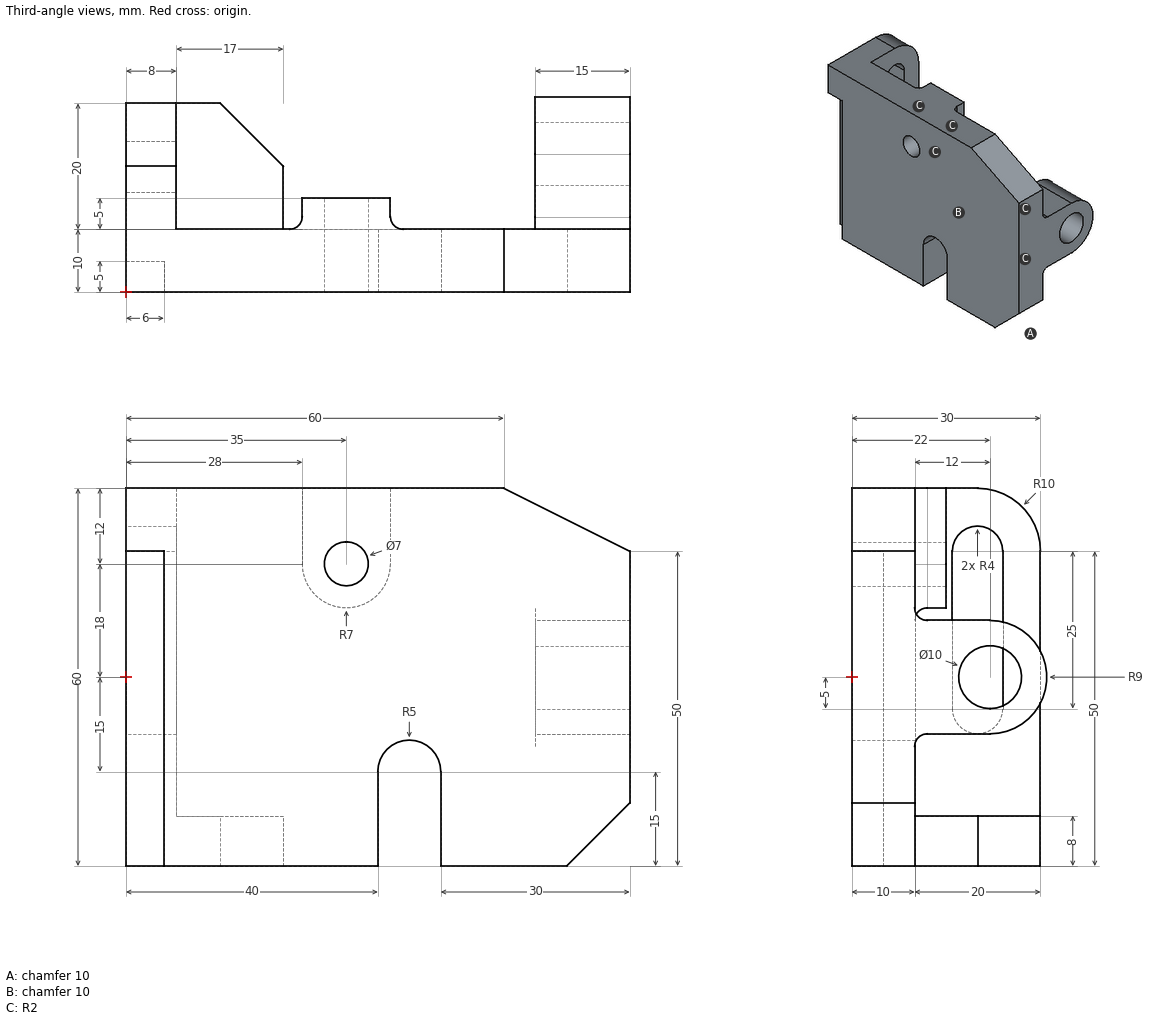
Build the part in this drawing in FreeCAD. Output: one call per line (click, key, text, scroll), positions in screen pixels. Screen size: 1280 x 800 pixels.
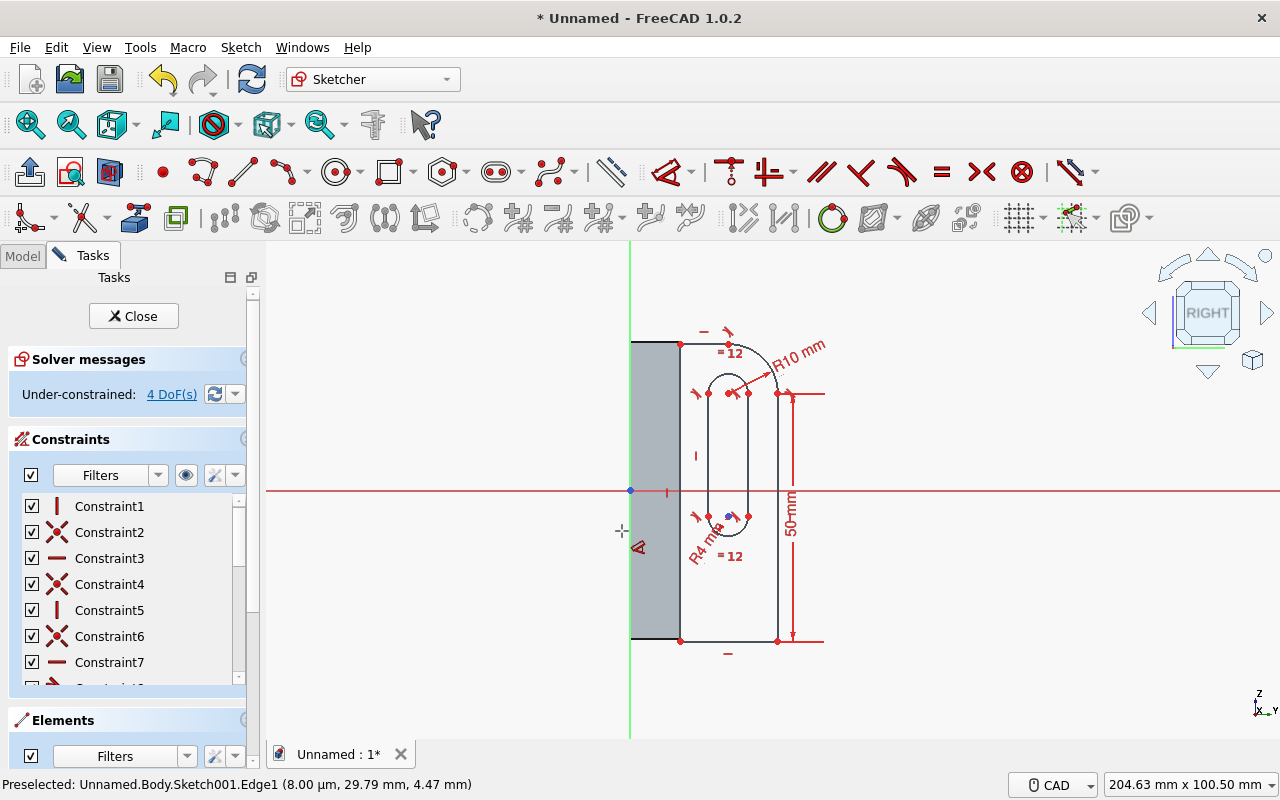
click(749, 642)
click(729, 676)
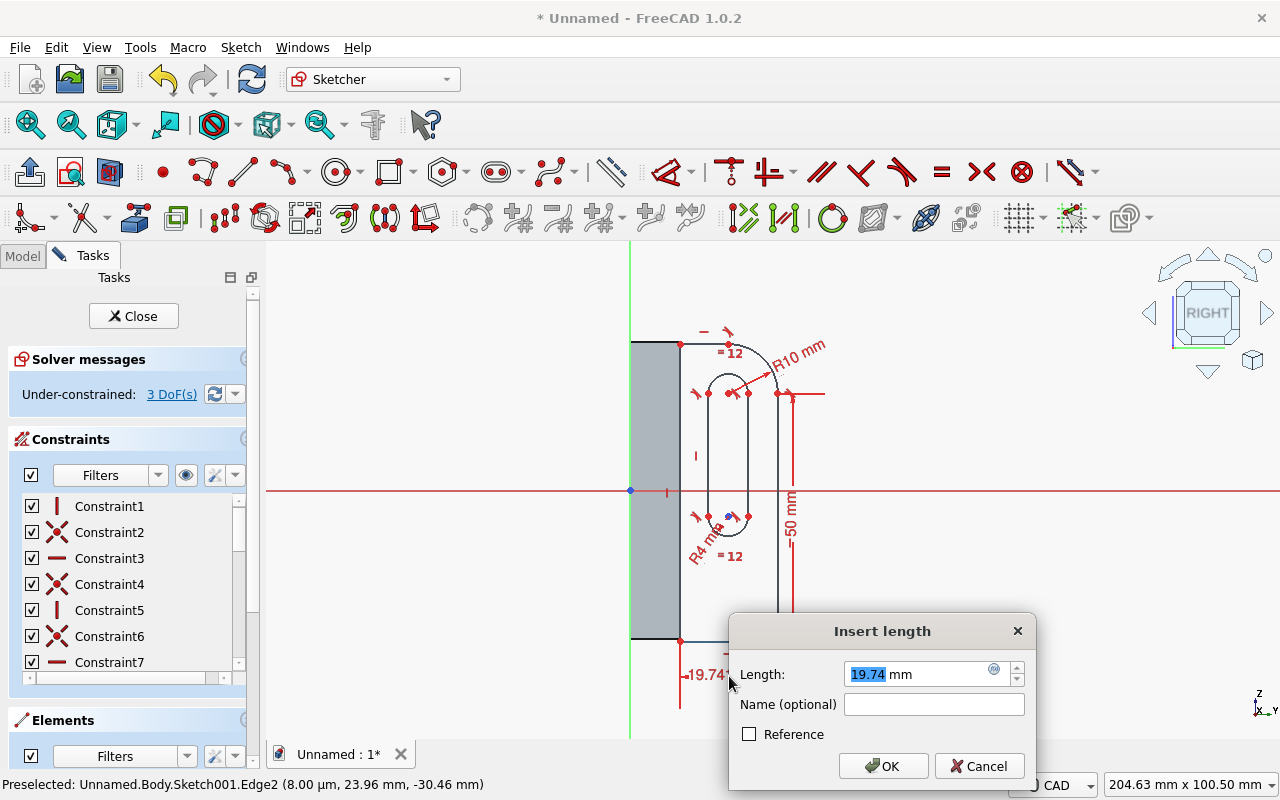
text(20)
key(Return)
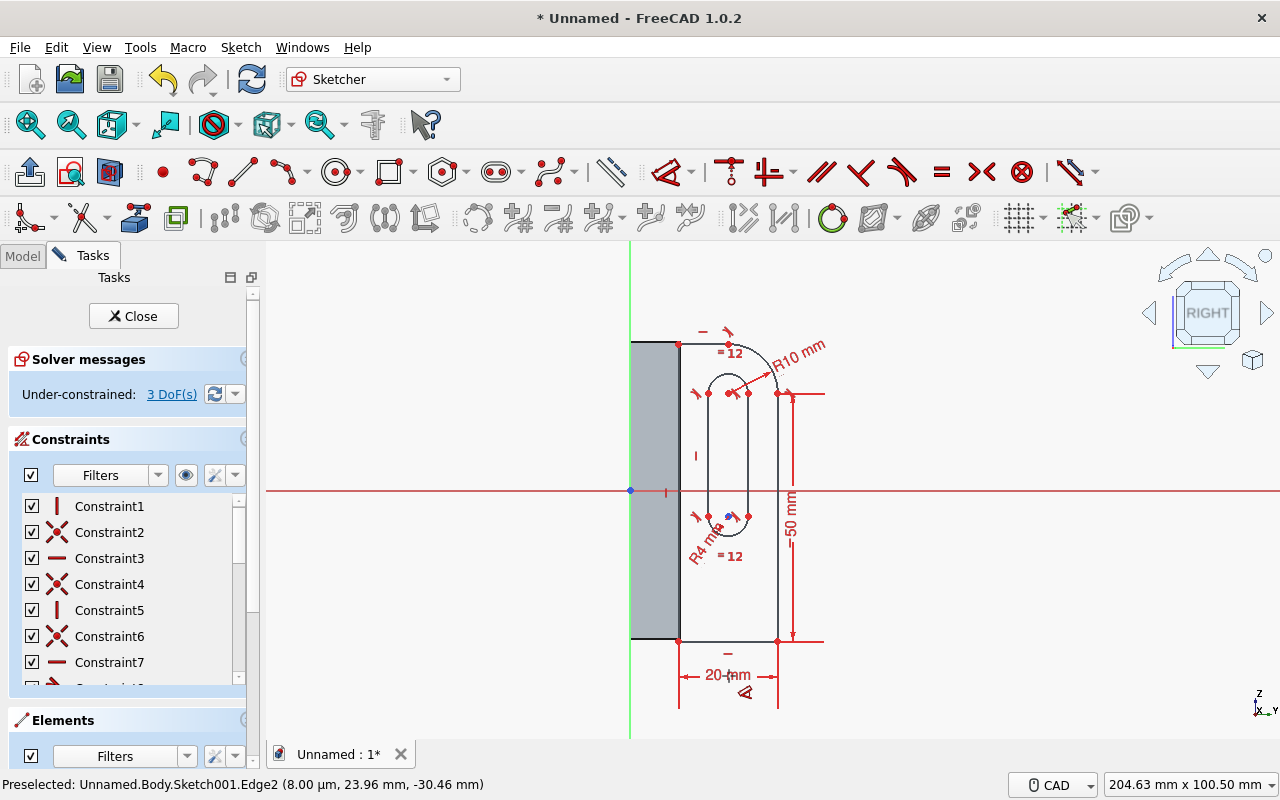
scroll(708, 480, up, 2)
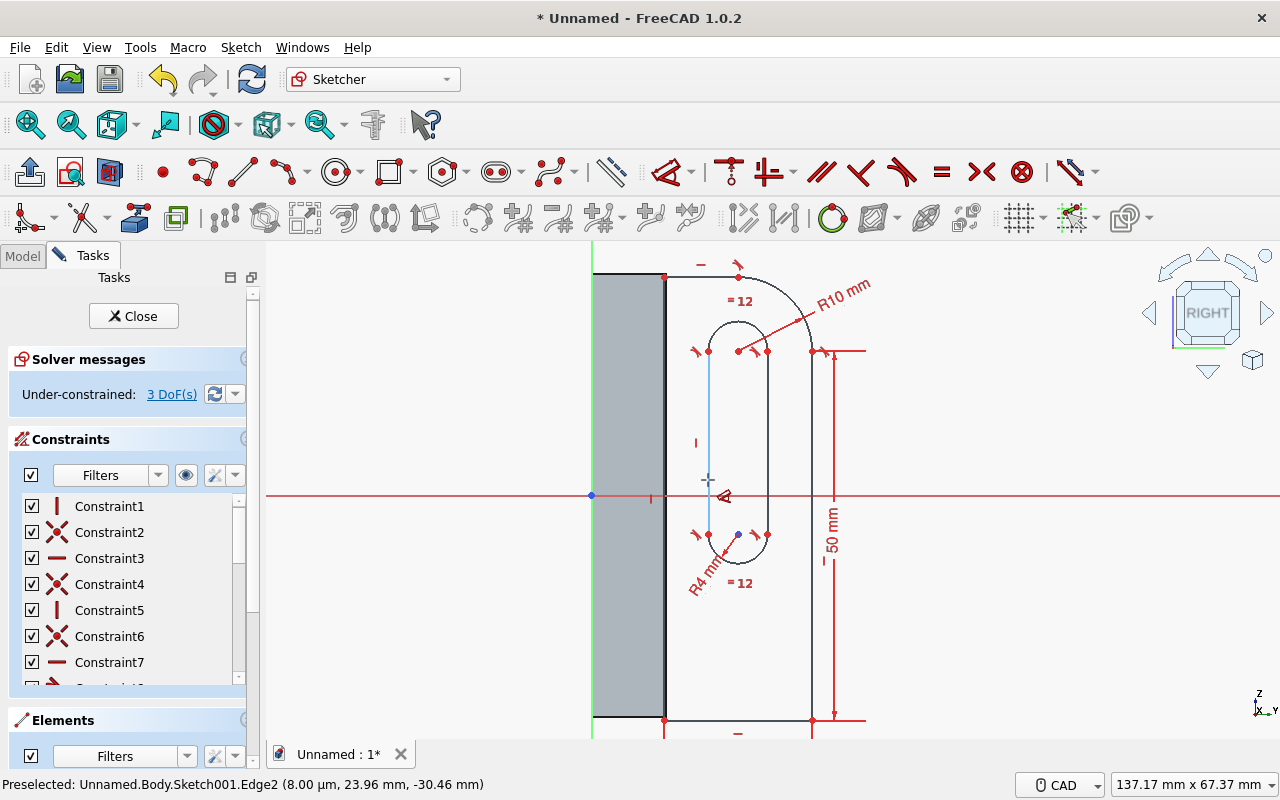
click(709, 479)
click(743, 443)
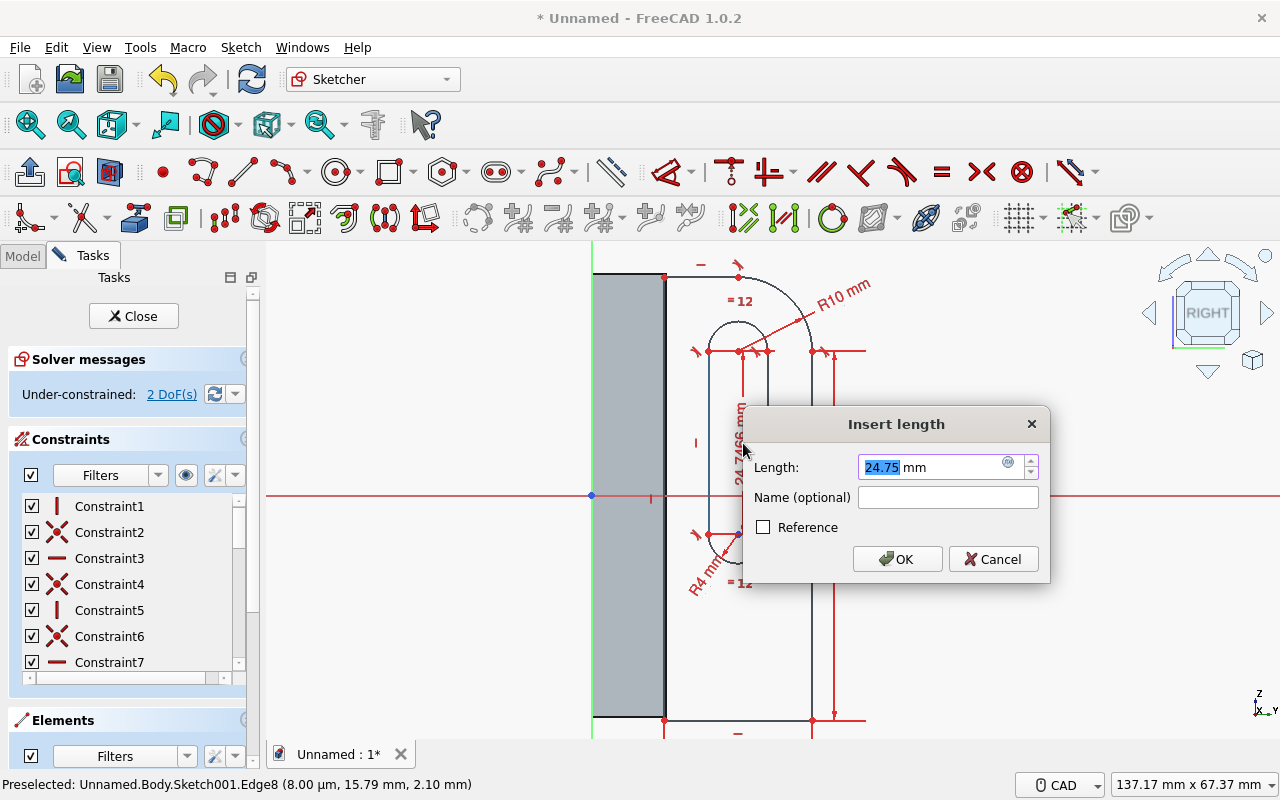
text(25)
key(Return)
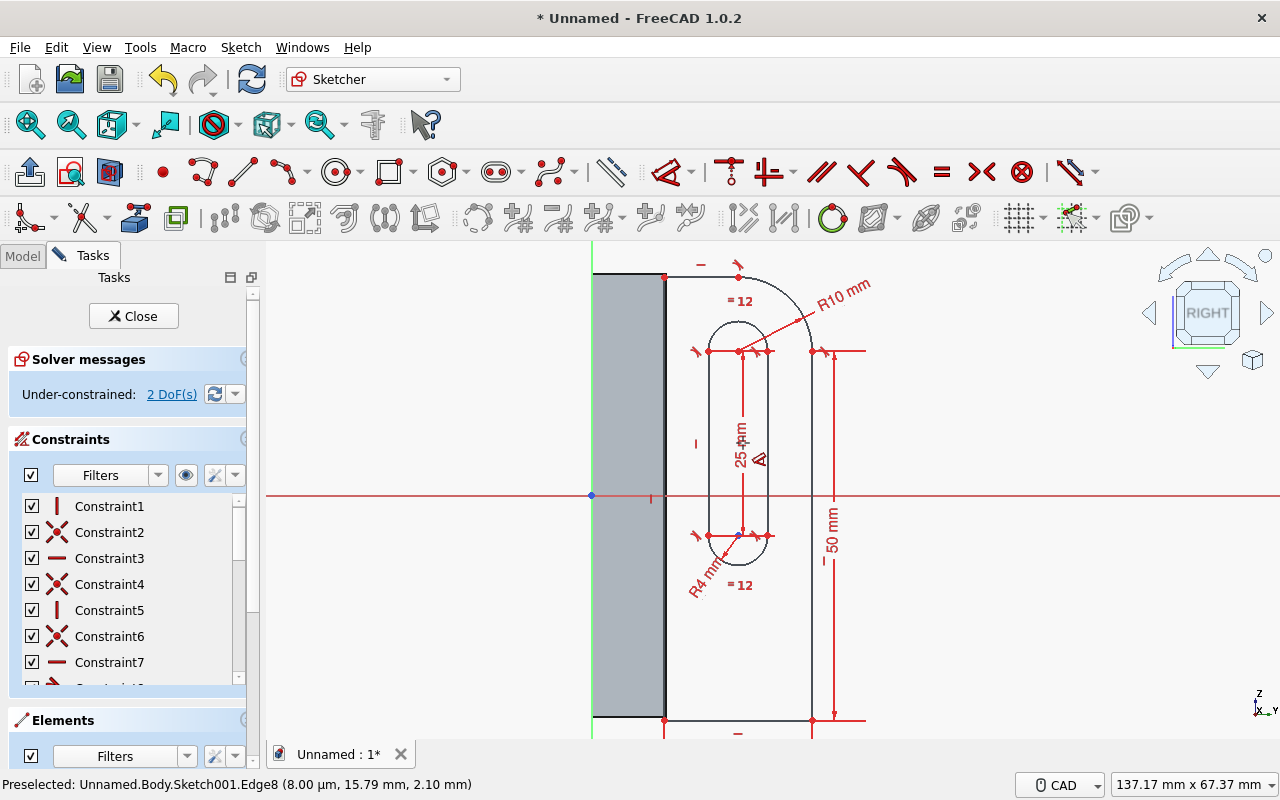
click(709, 536)
click(558, 516)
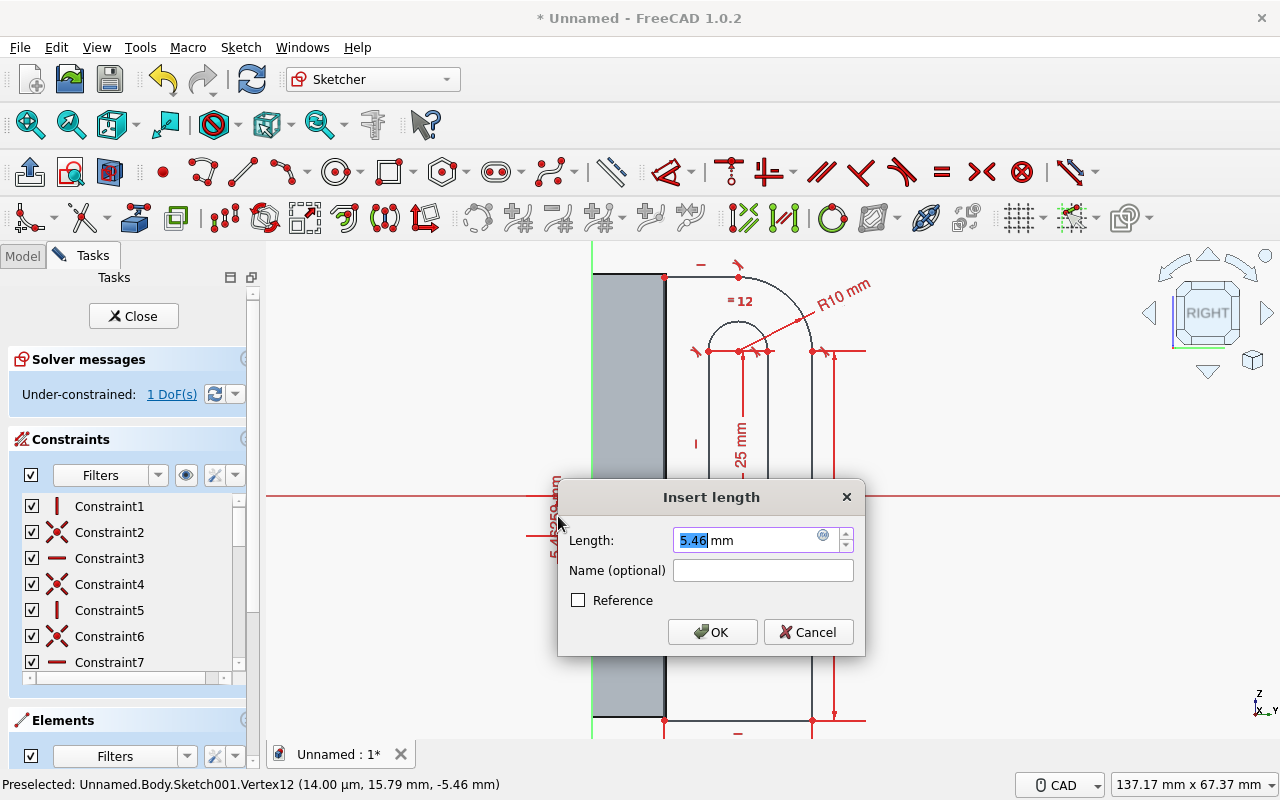
text(5)
key(Return)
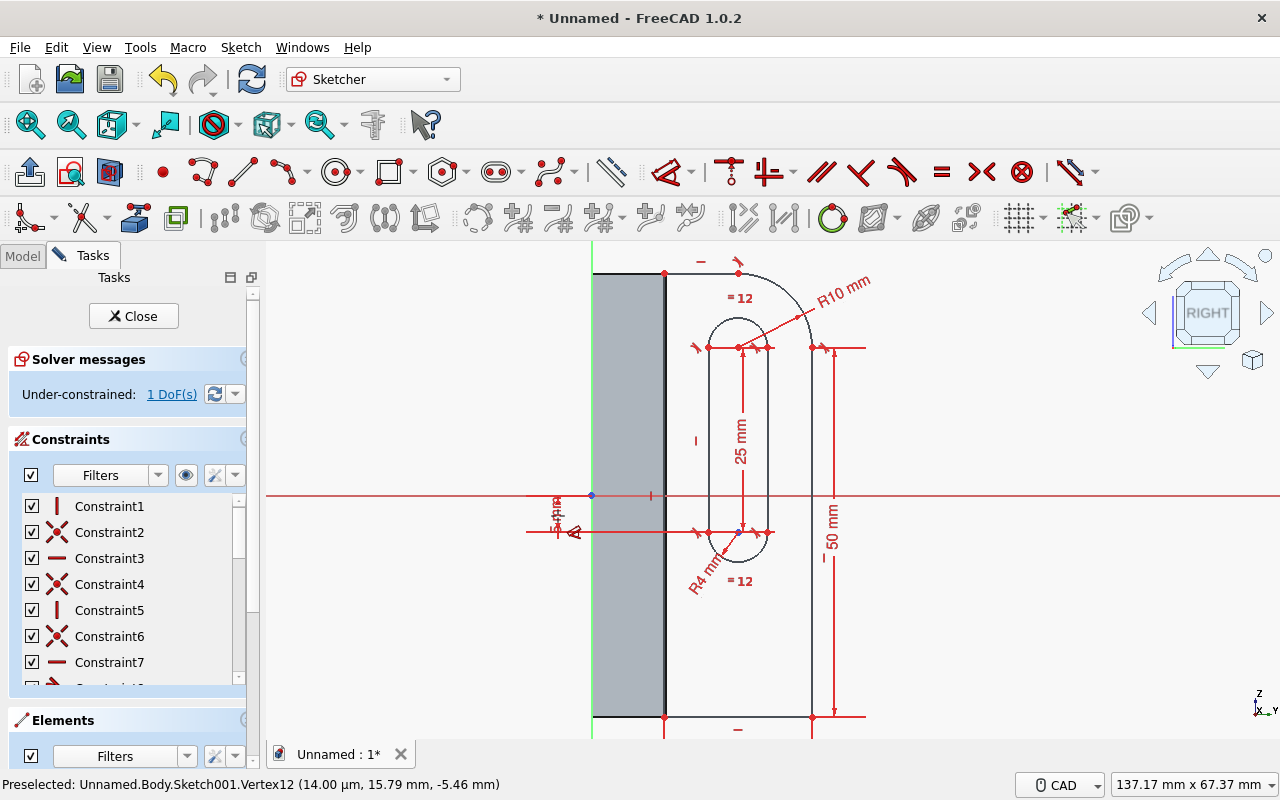
click(812, 348)
click(702, 314)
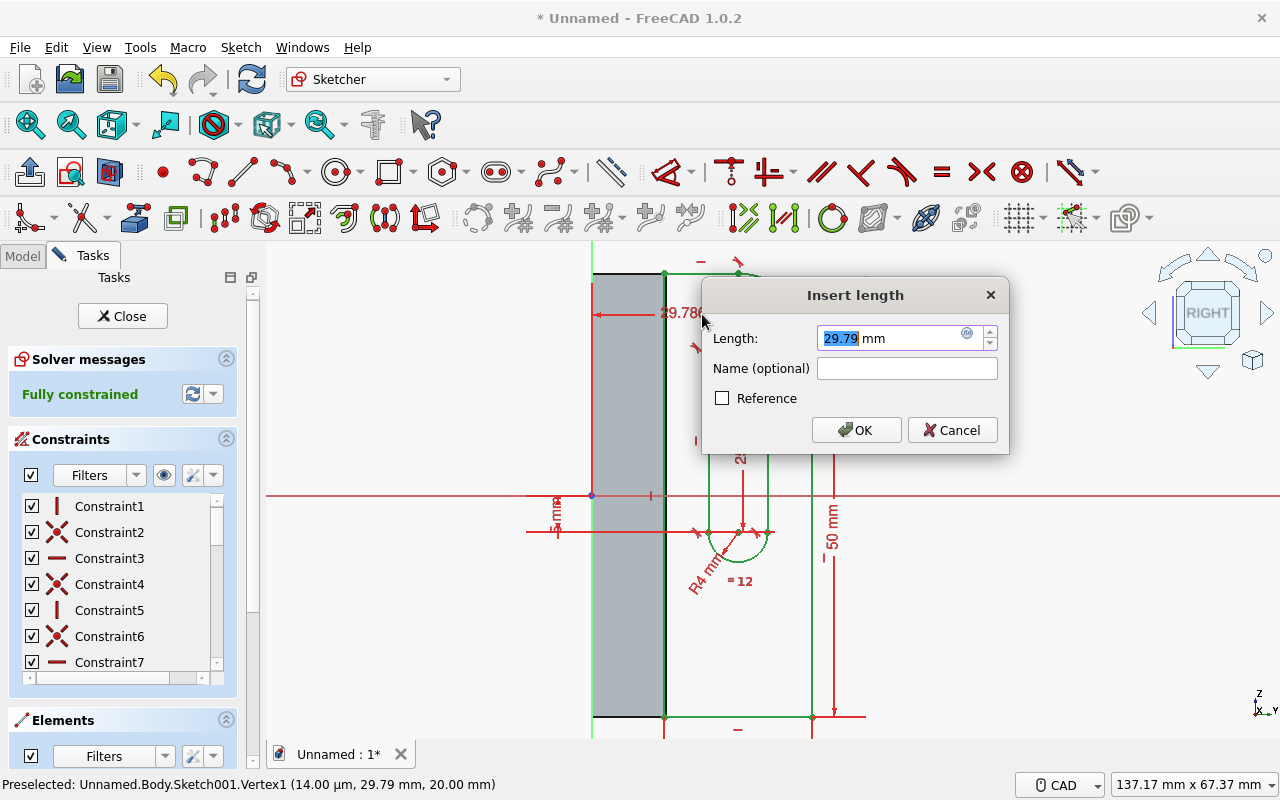
text(30)
key(Return)
key(Escape)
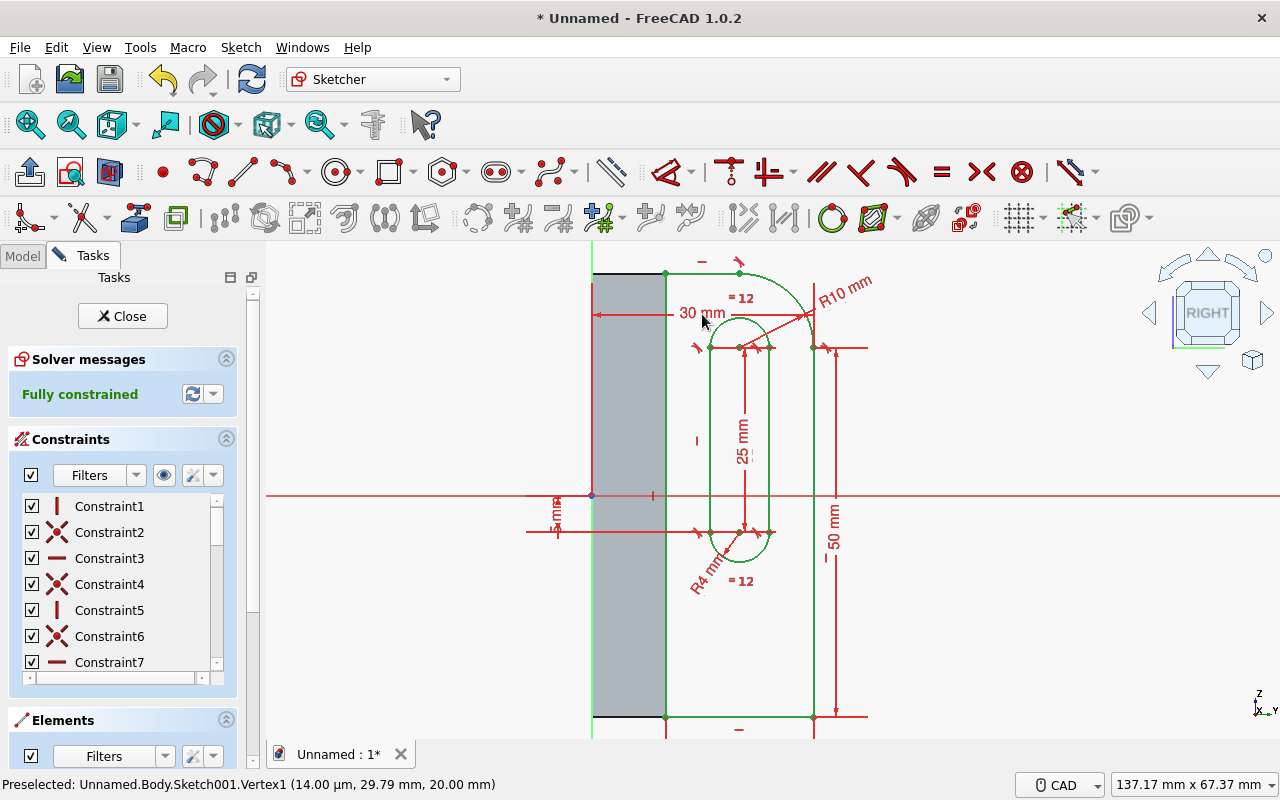
click(123, 316)